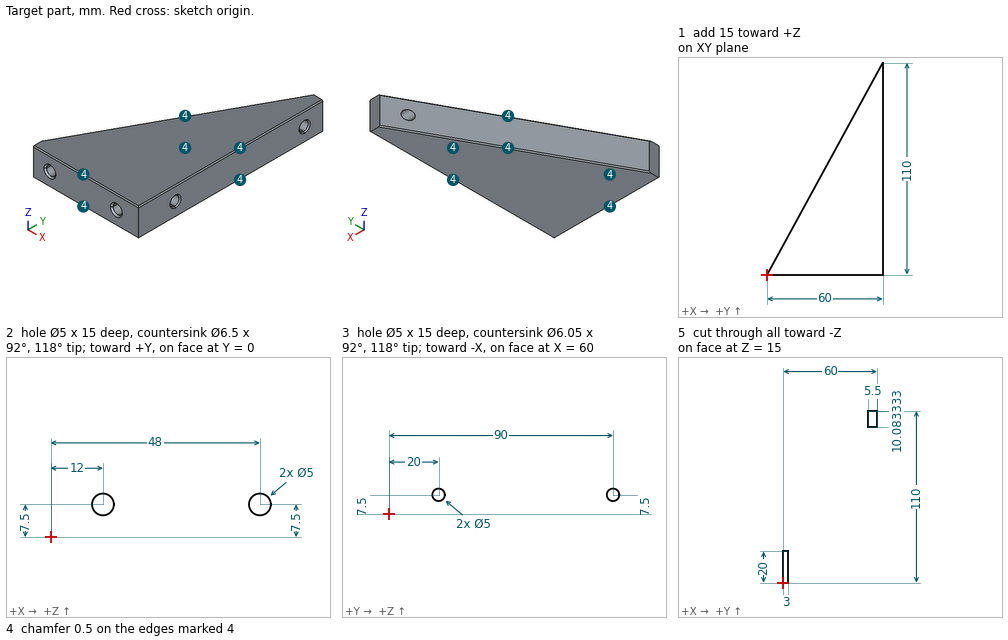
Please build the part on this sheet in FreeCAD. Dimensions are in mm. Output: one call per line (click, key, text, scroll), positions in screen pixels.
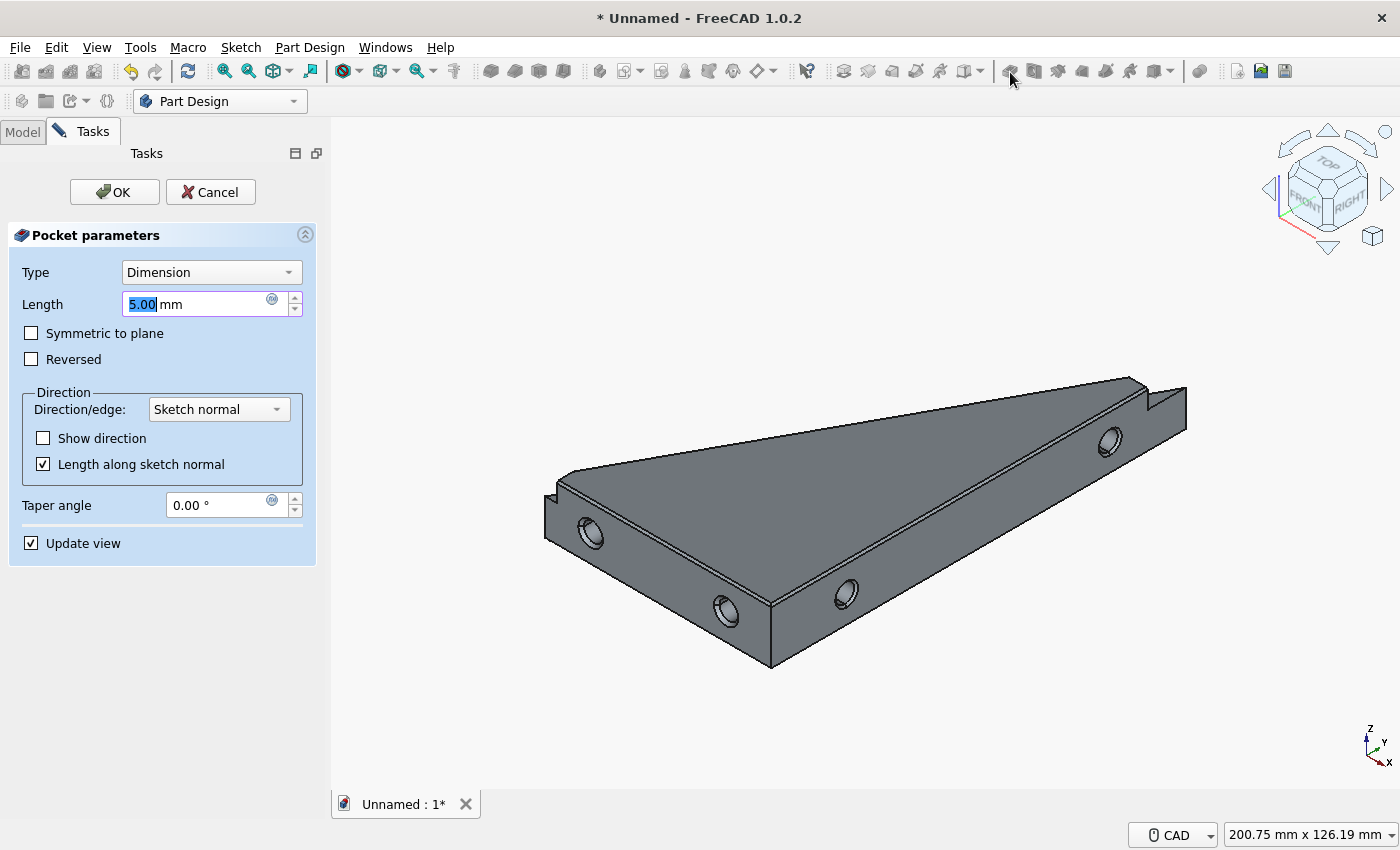
click(212, 272)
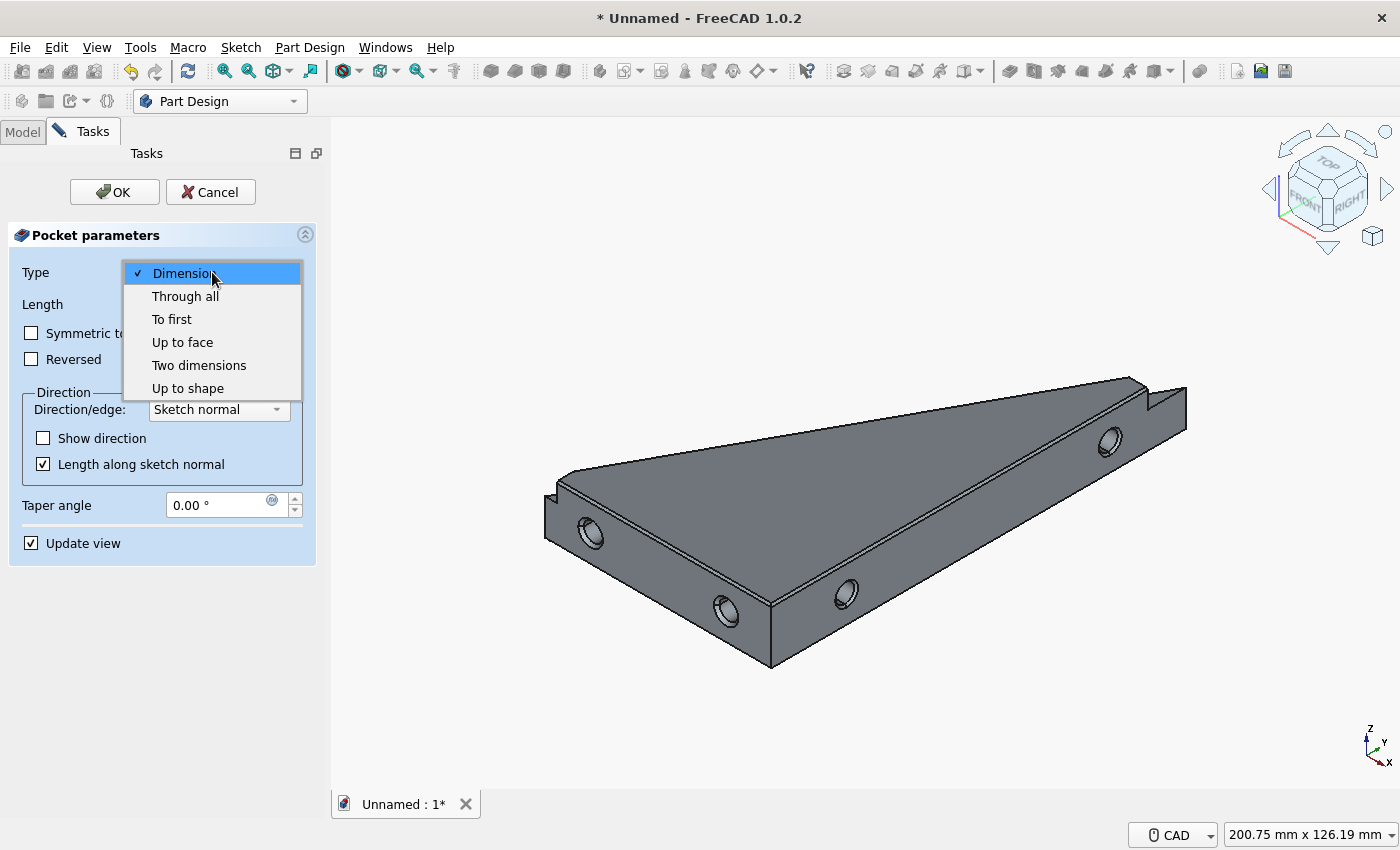
click(212, 296)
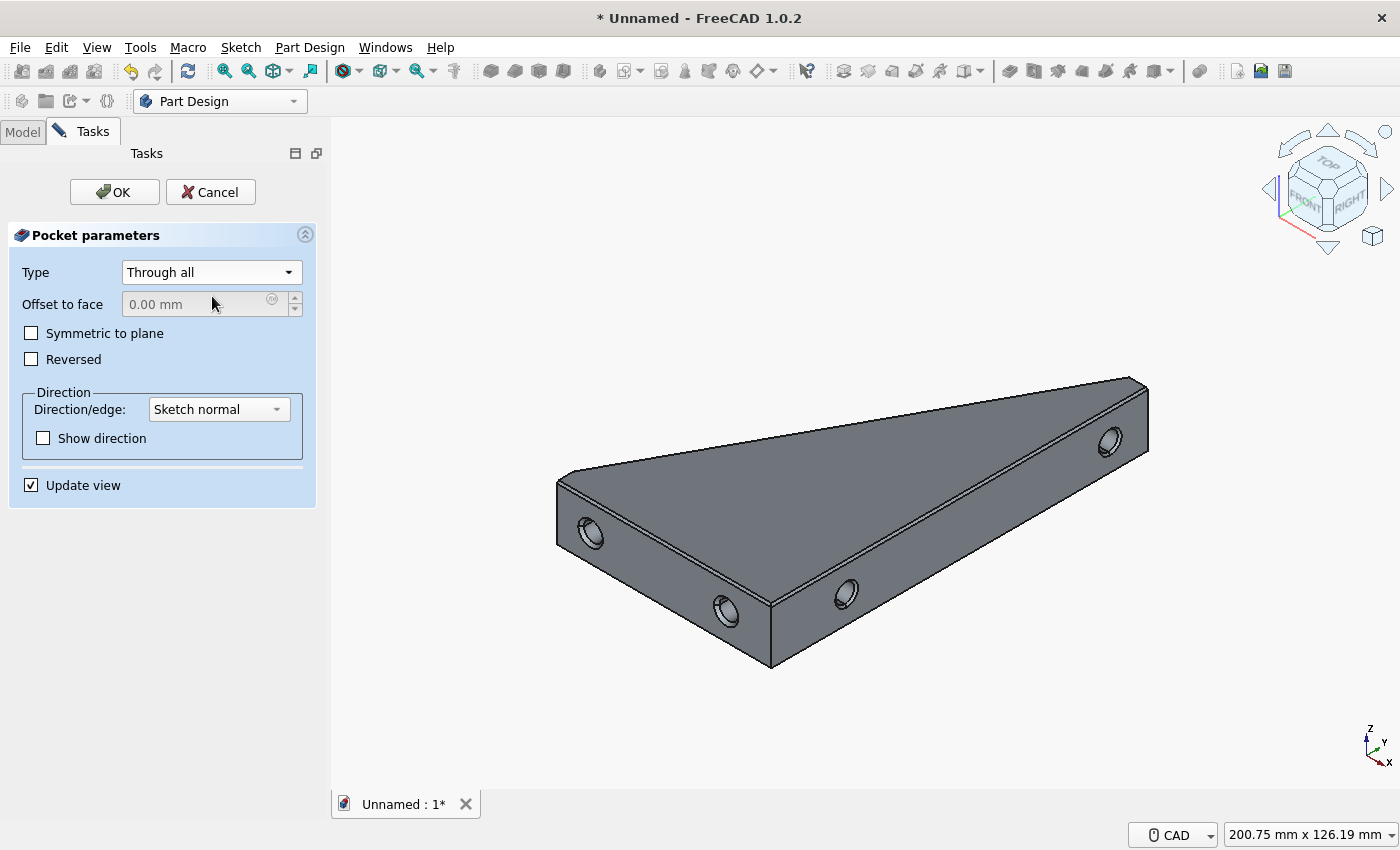
click(115, 192)